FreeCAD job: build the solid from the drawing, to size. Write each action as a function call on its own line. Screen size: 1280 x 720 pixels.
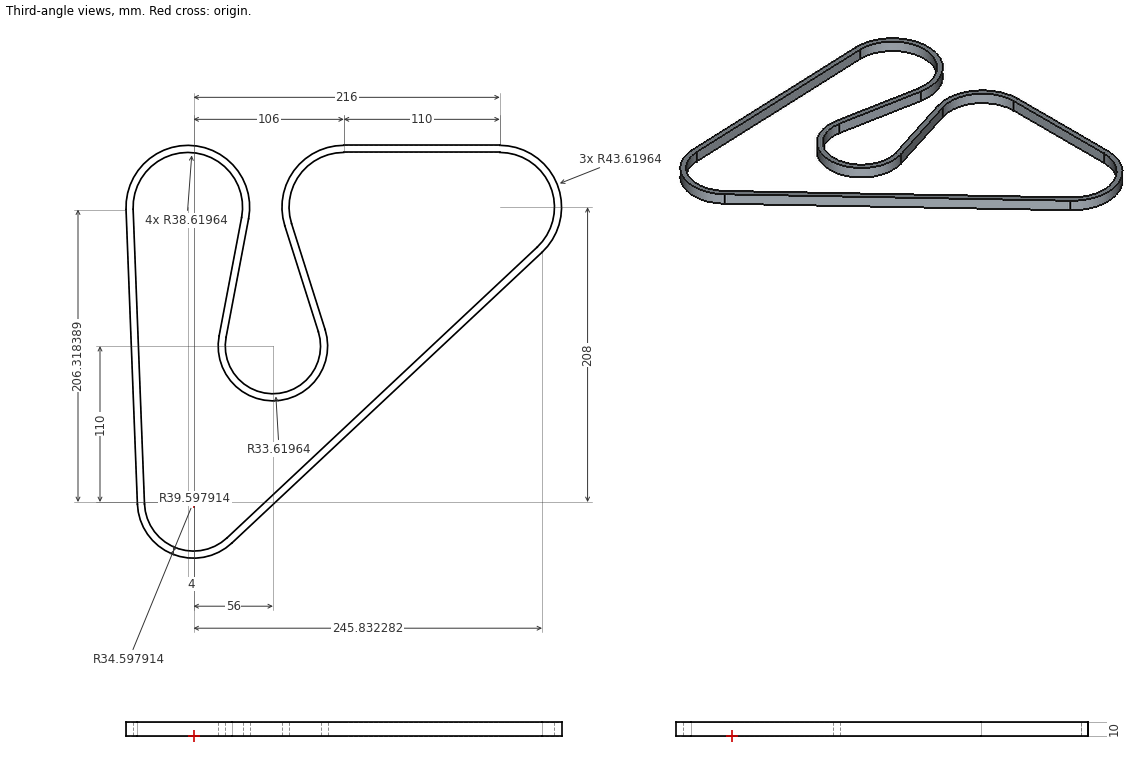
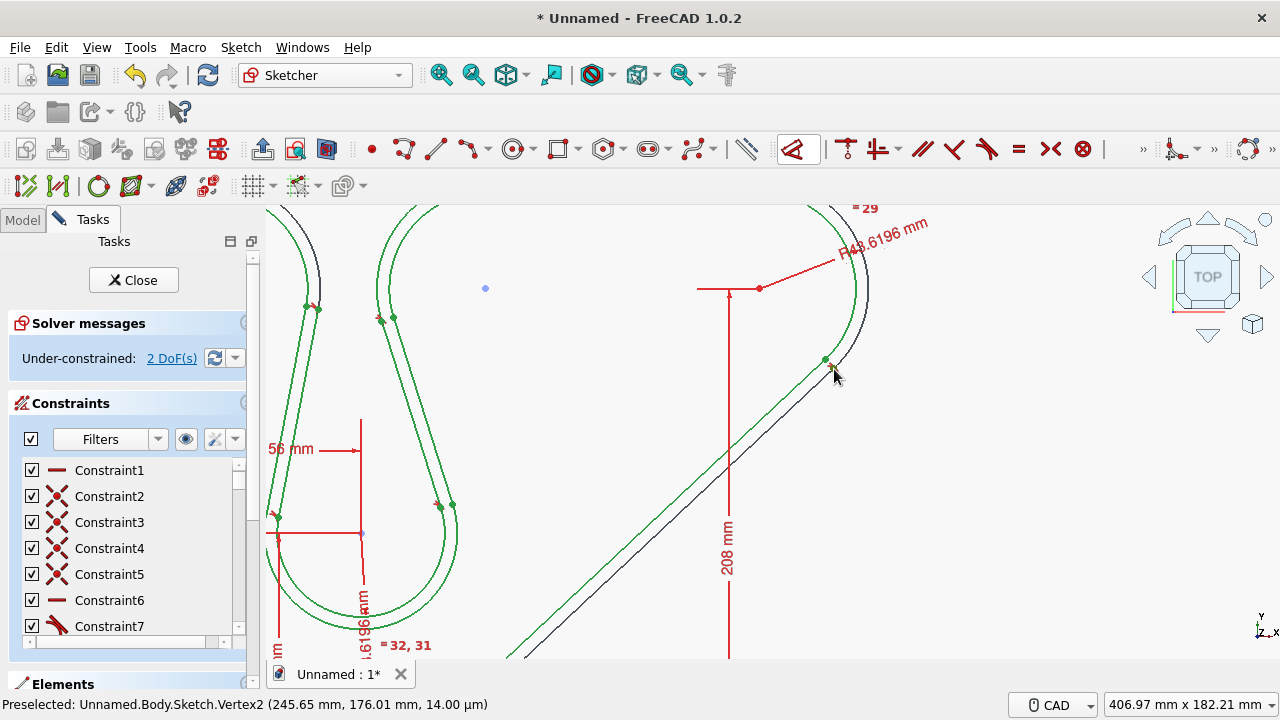
key(l)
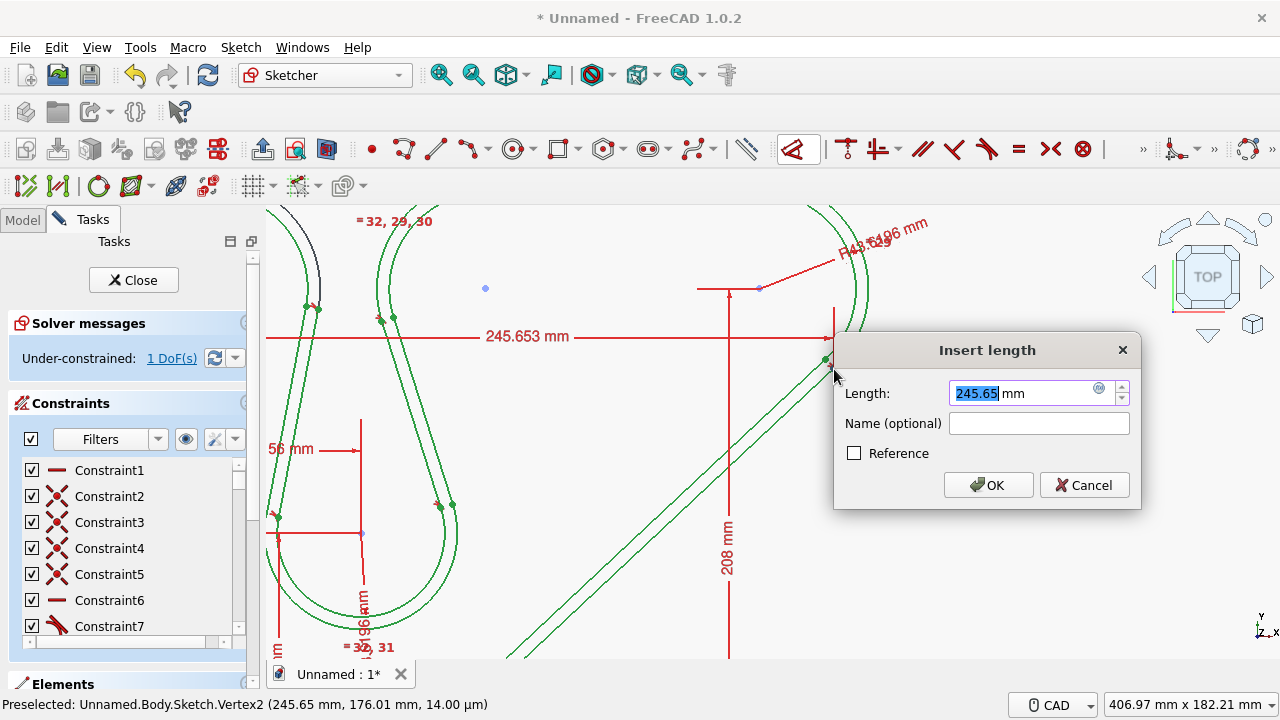
text(245.832282)
key(Return)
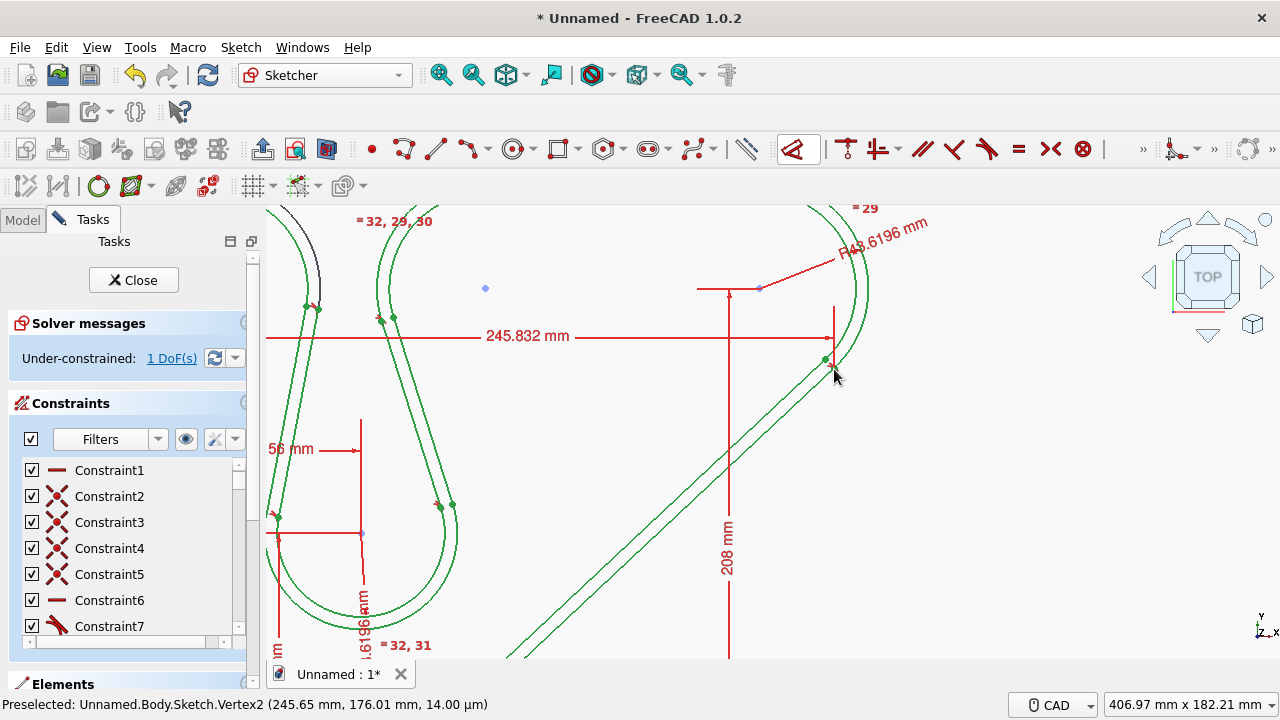
scroll(834, 370, down, 5)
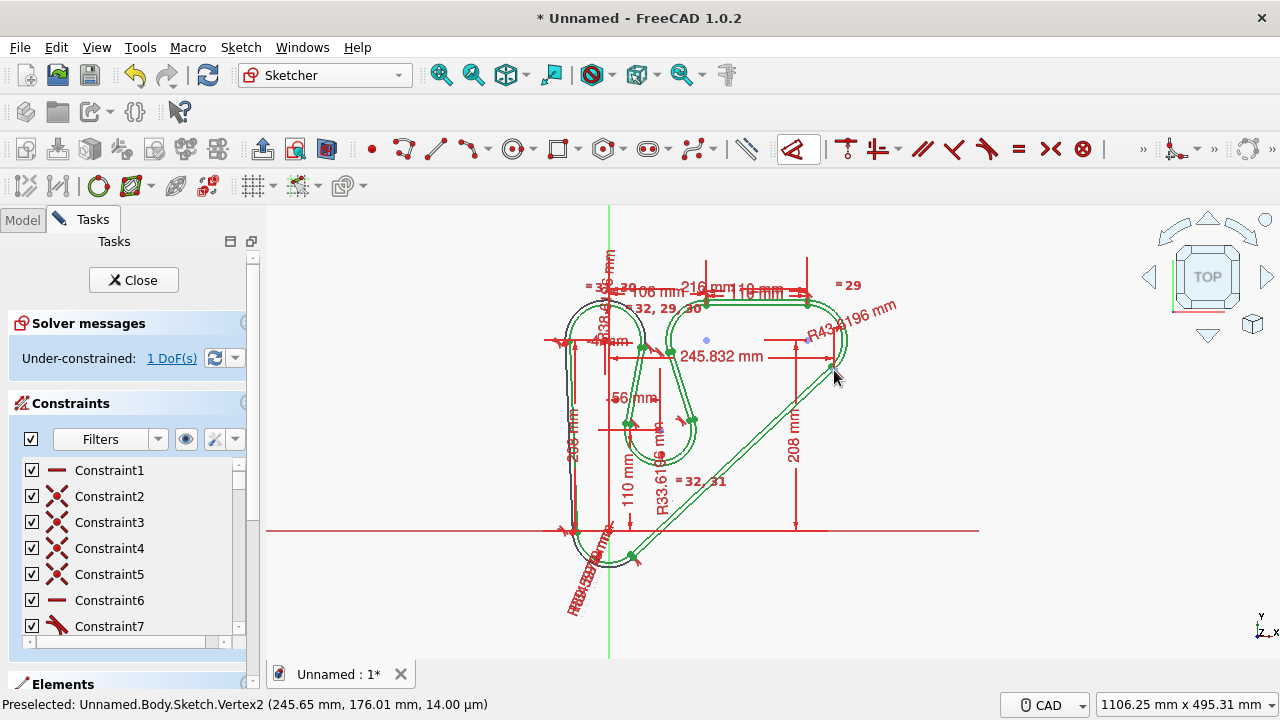
scroll(565, 343, up, 5)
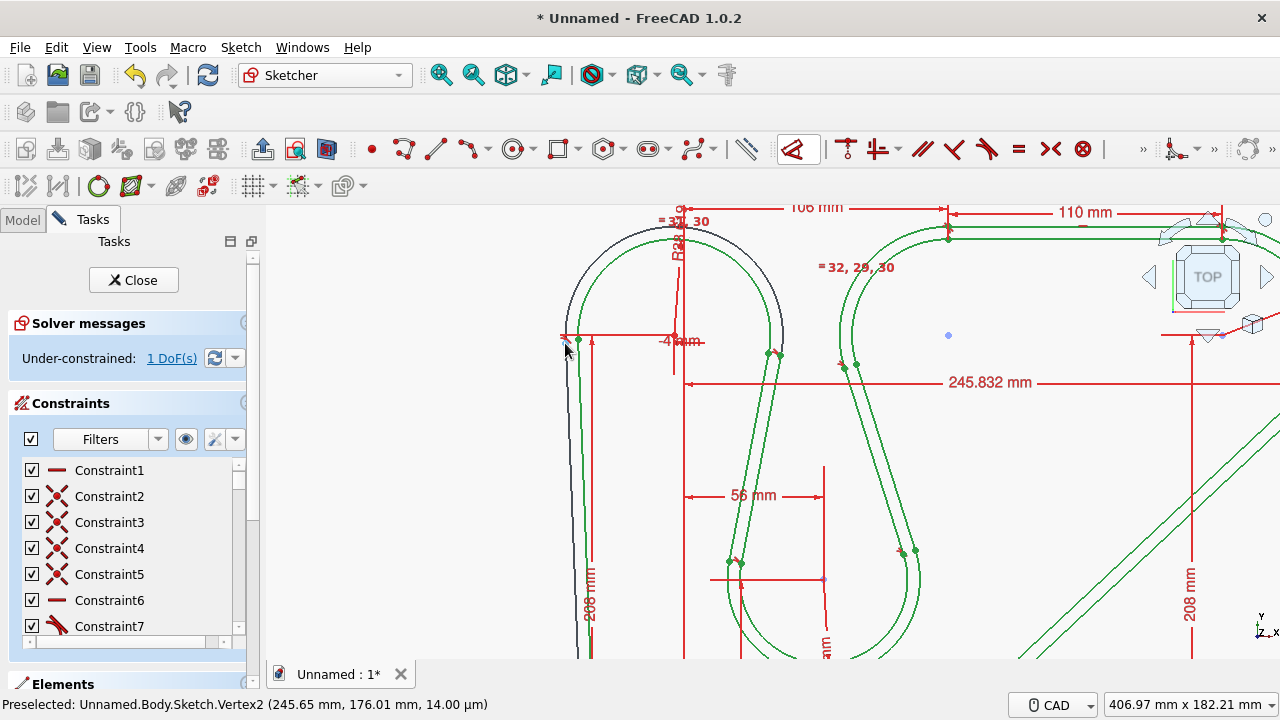
click(566, 343)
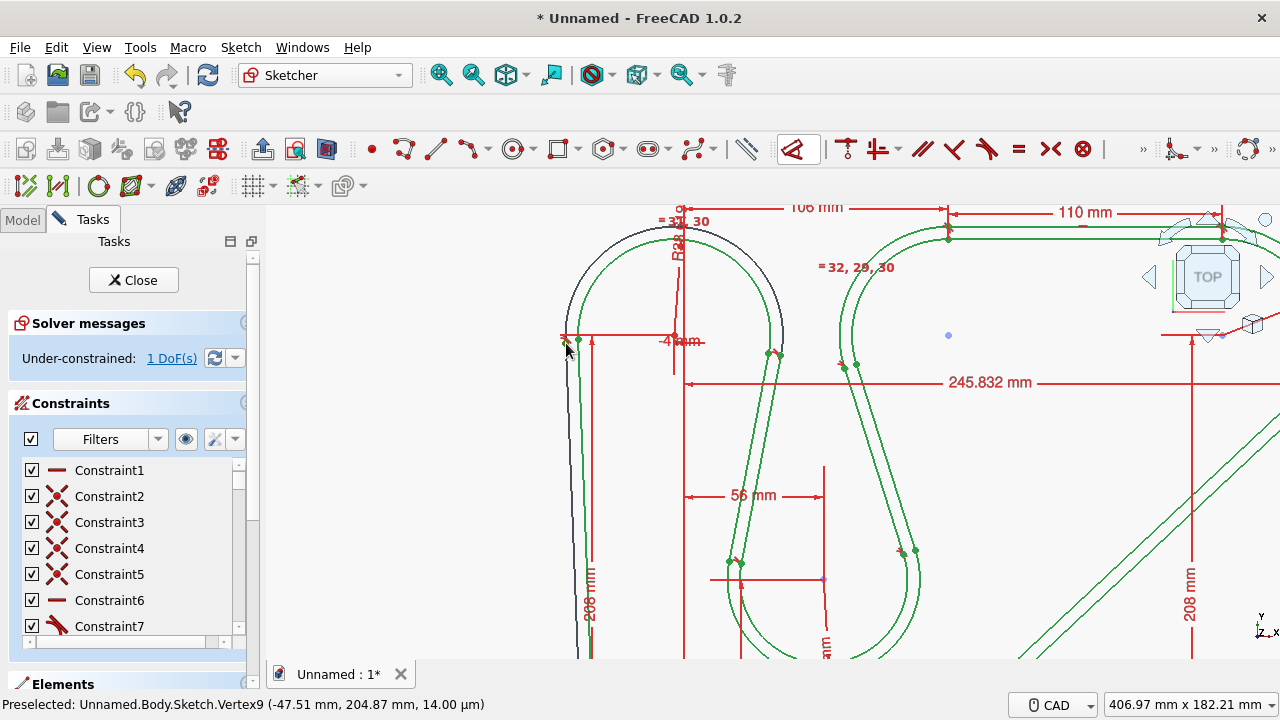
click(814, 150)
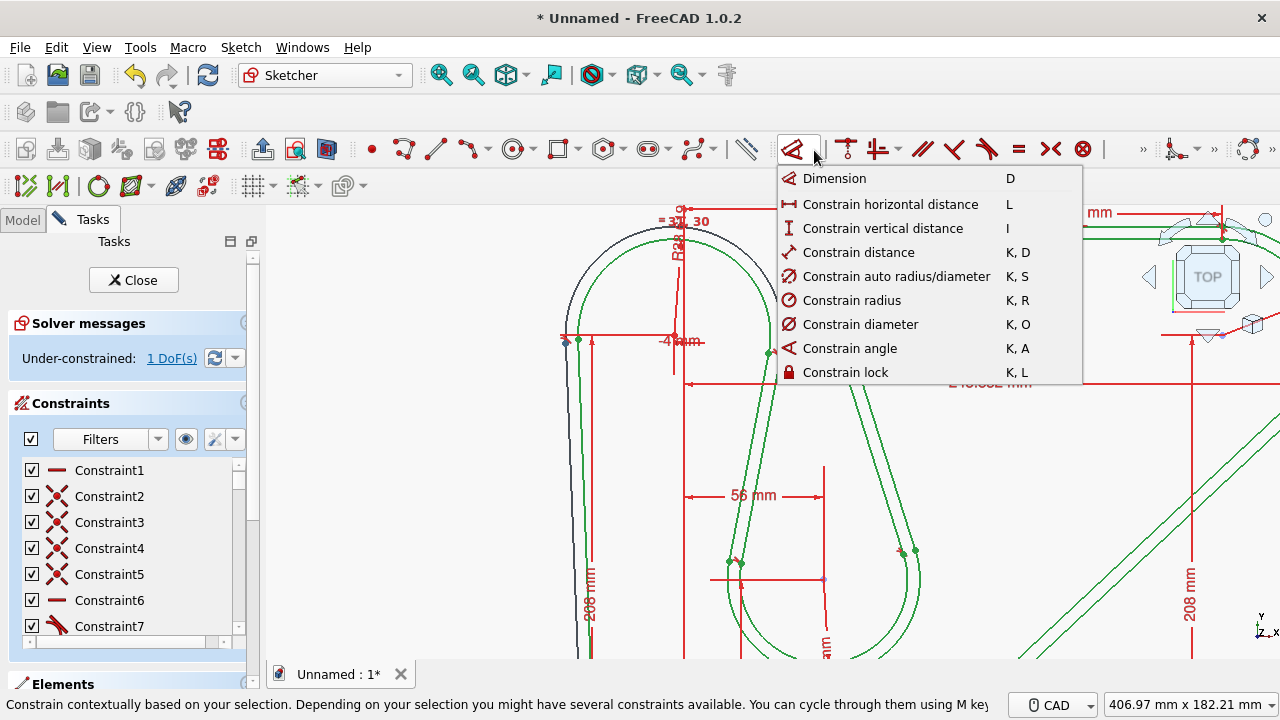
click(930, 228)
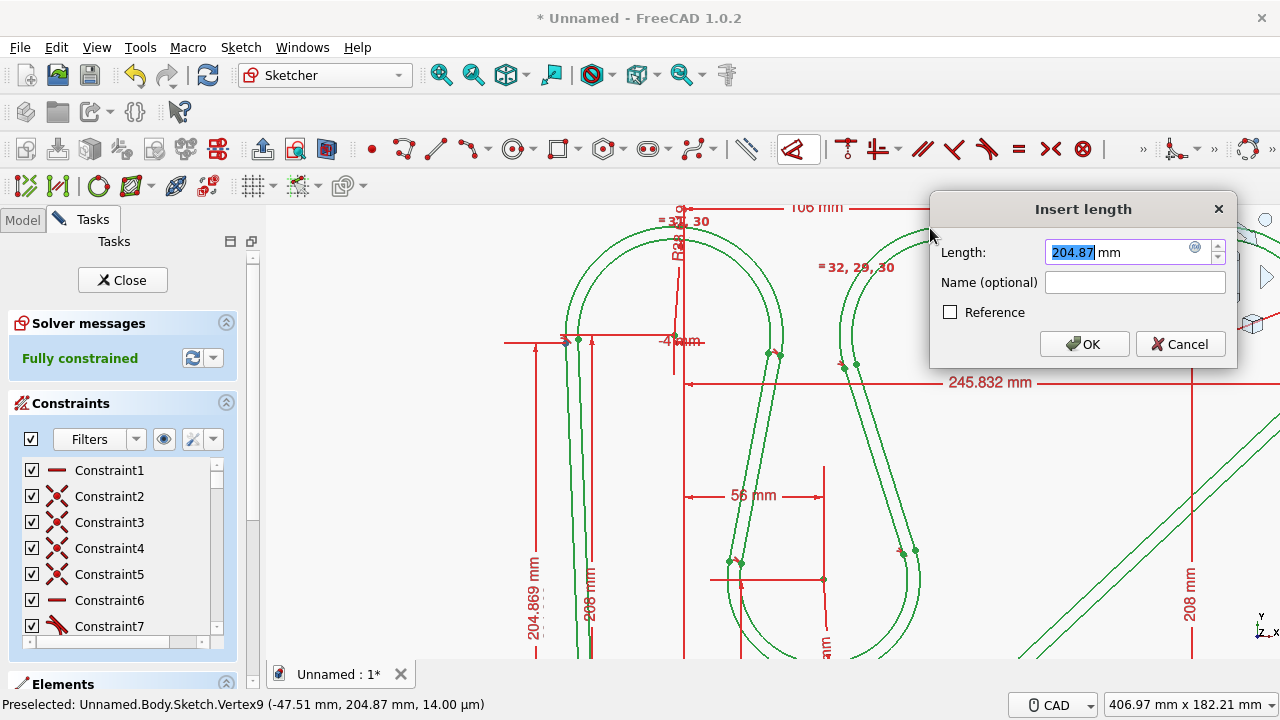
text(206.318389)
key(Return)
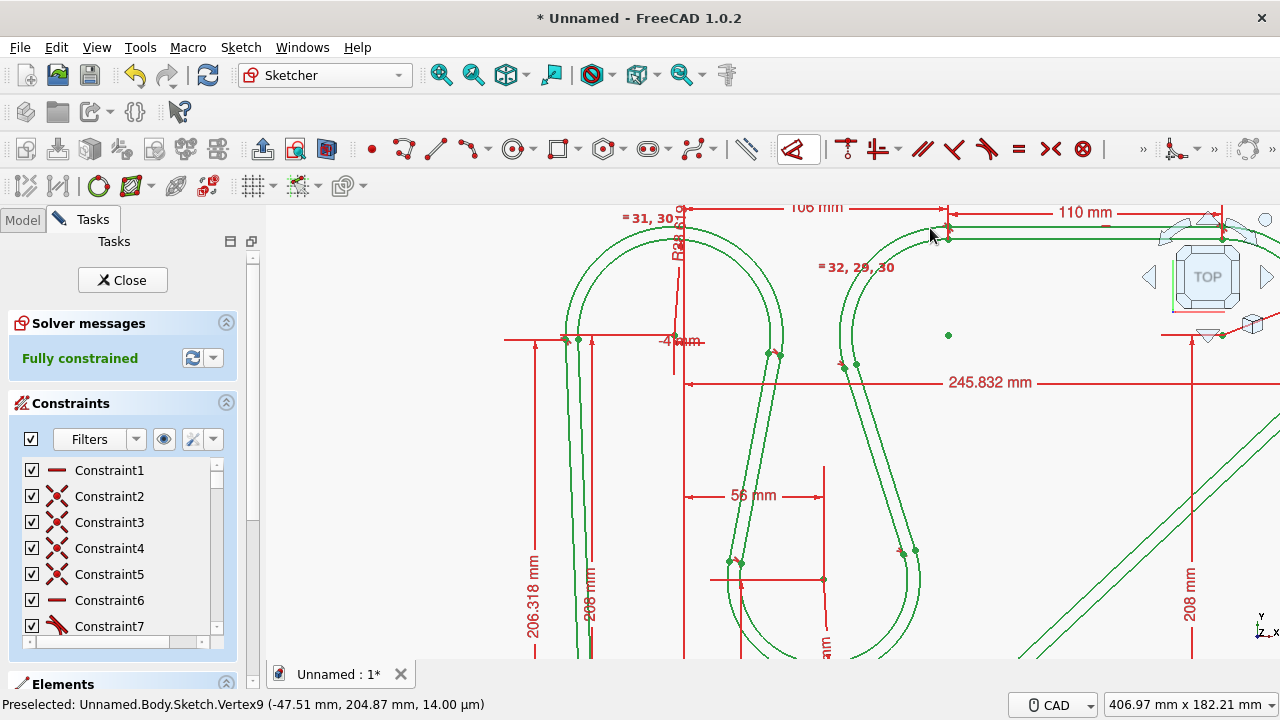
click(123, 280)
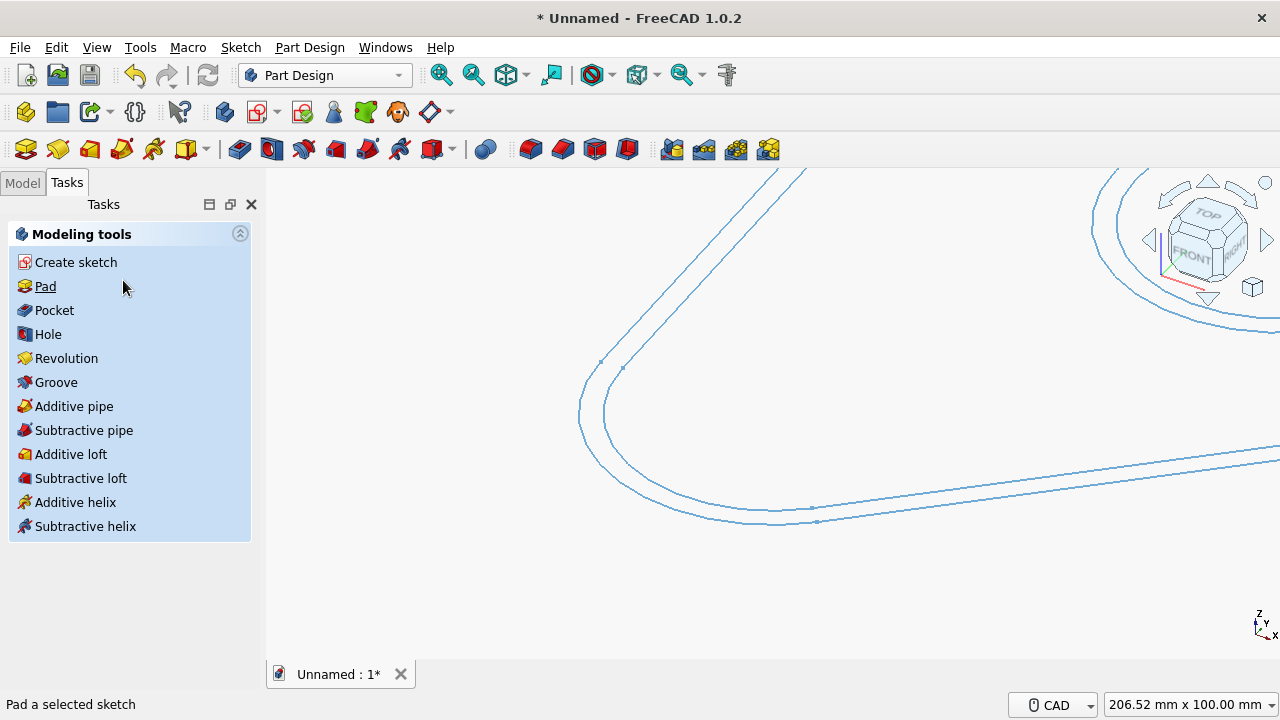
click(26, 150)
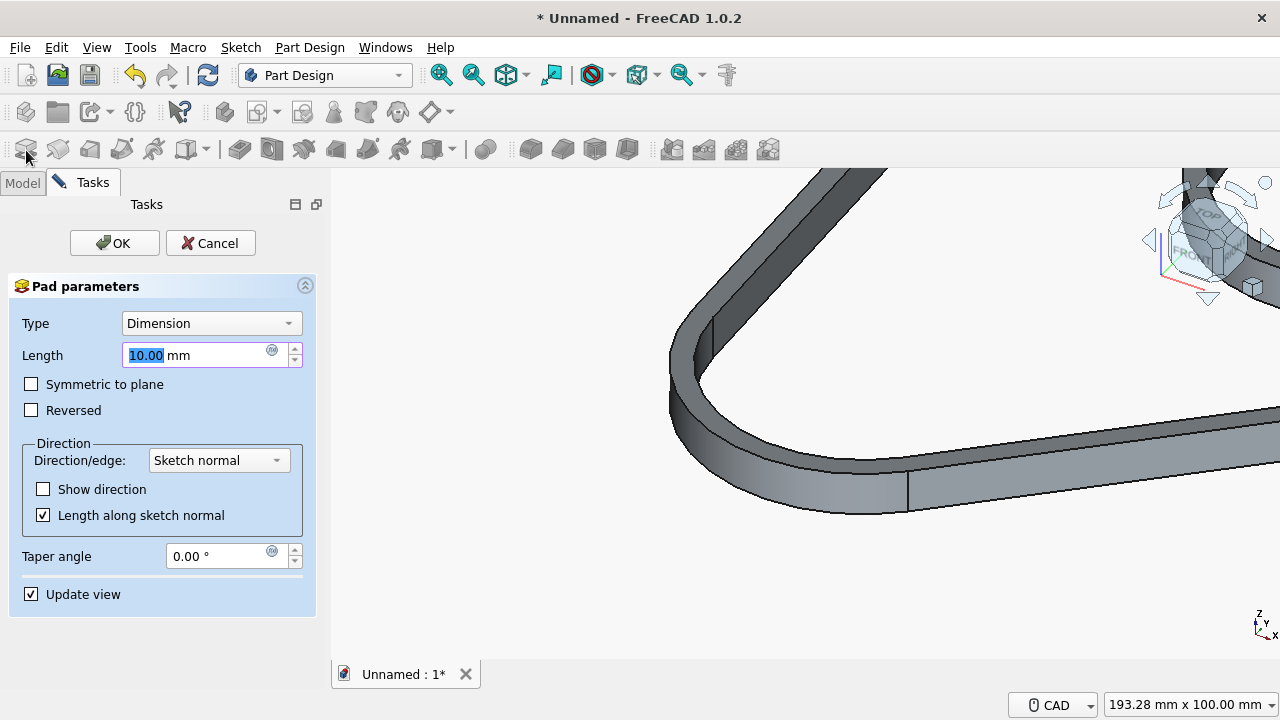
text(10)
key(Tab)